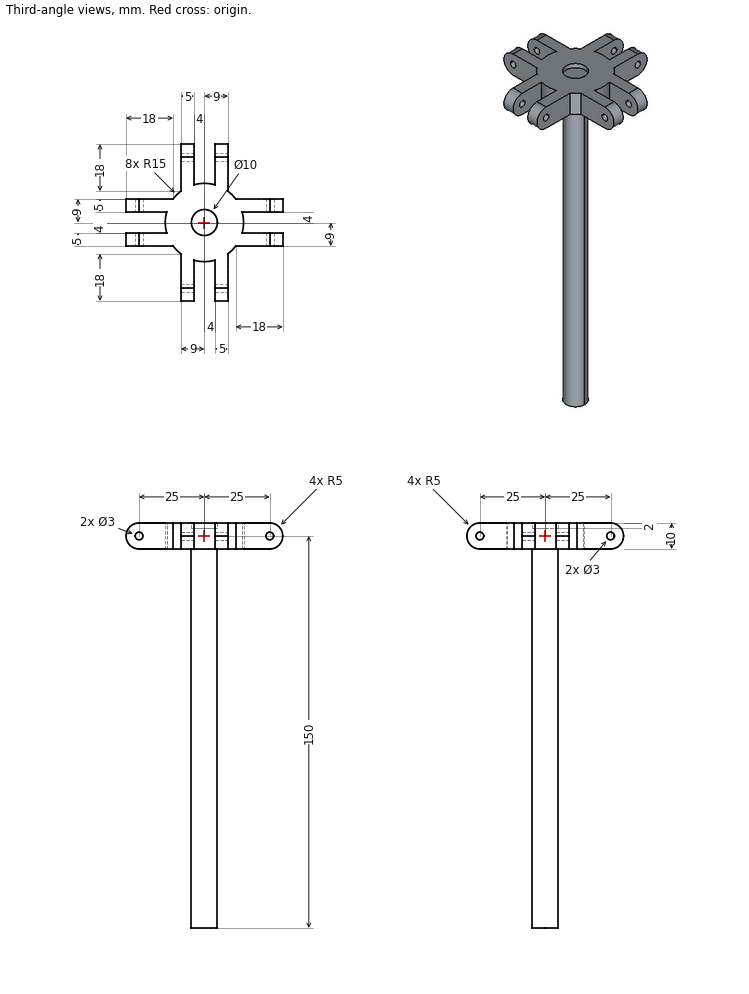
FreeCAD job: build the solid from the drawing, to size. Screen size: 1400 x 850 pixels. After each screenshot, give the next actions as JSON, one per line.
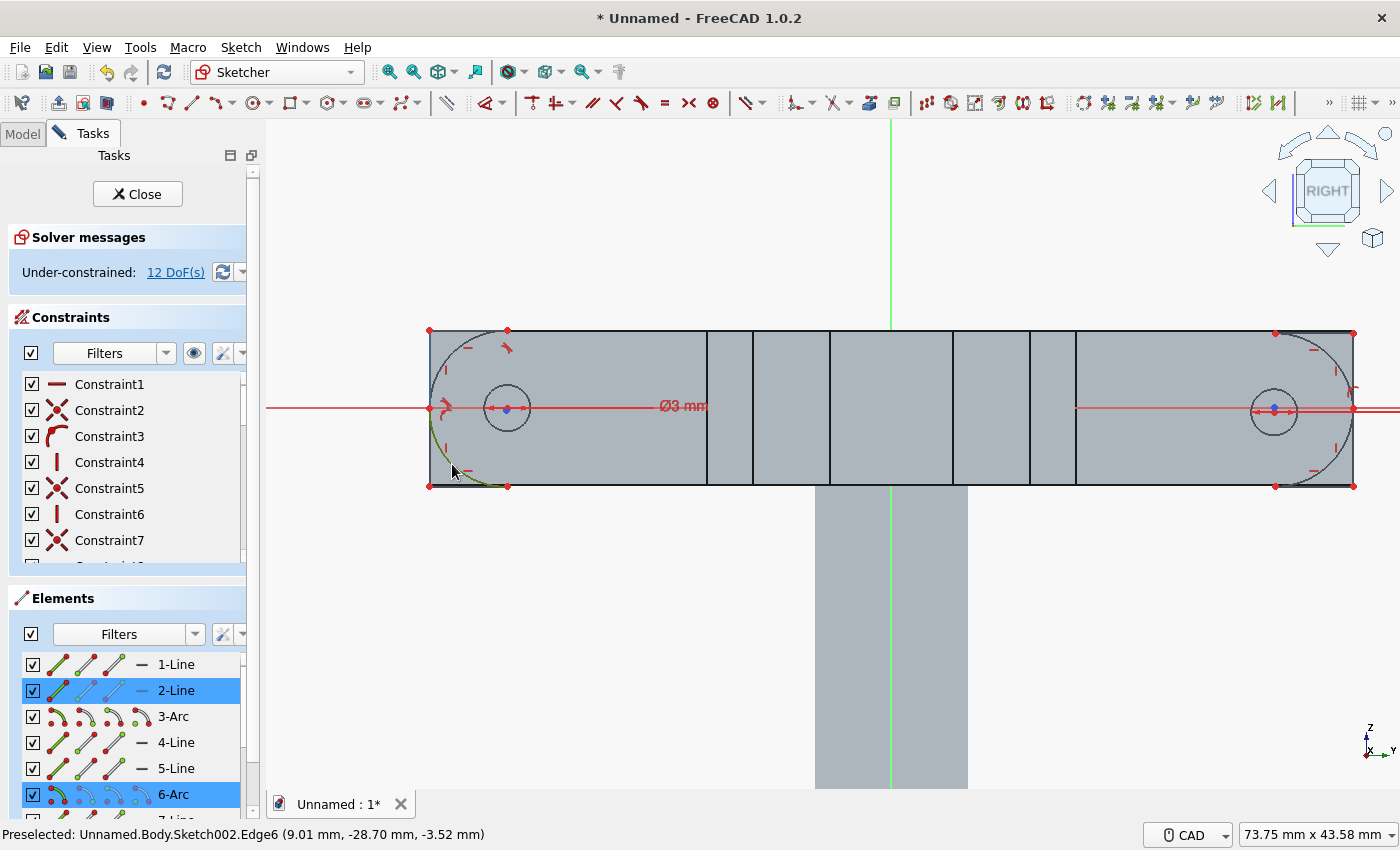
{"action": "key", "text": "t"}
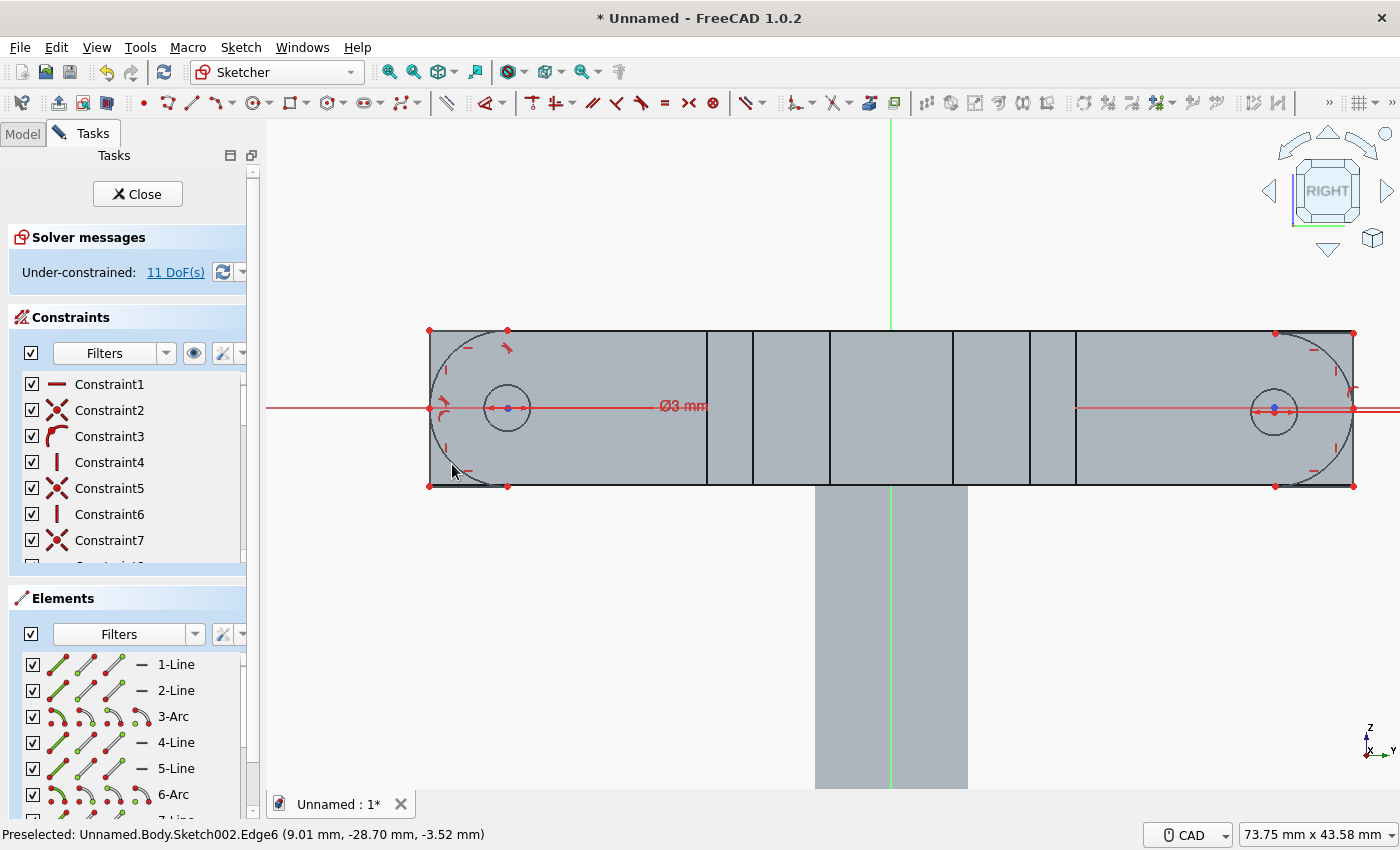
{"action": "left_click", "coordinate": [453, 487]}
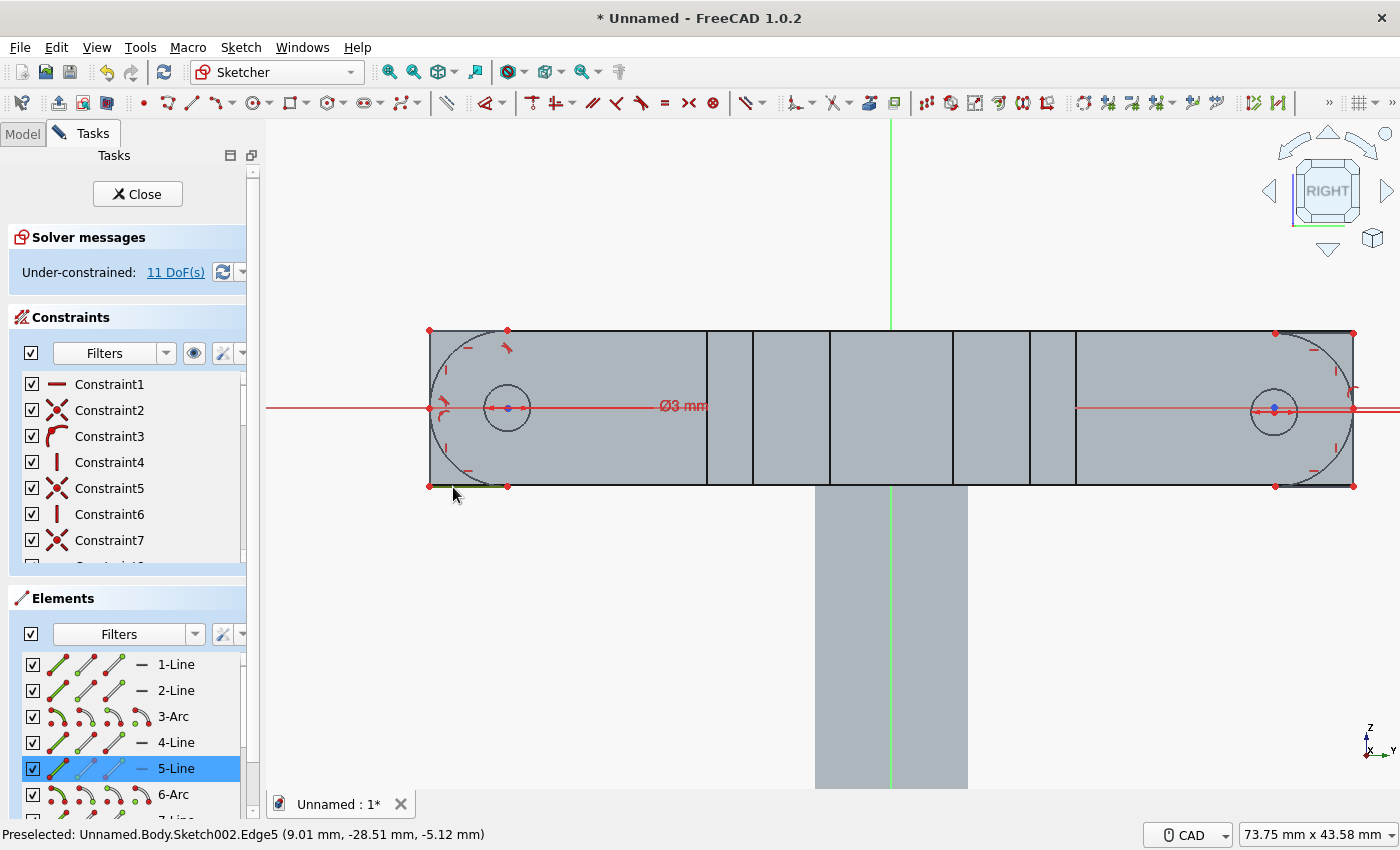
{"action": "left_click", "coordinate": [452, 463]}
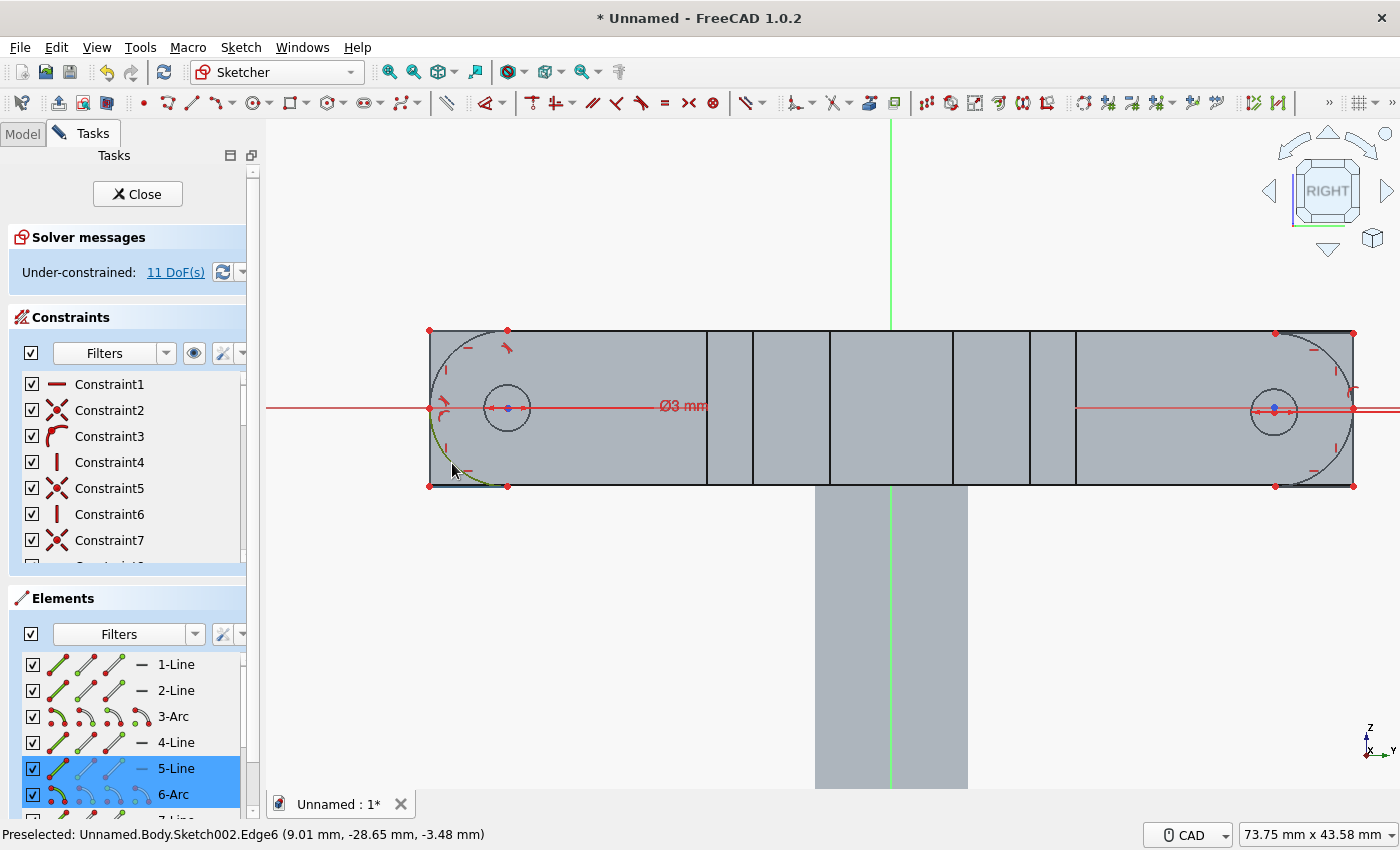
{"action": "left_click", "coordinate": [642, 104]}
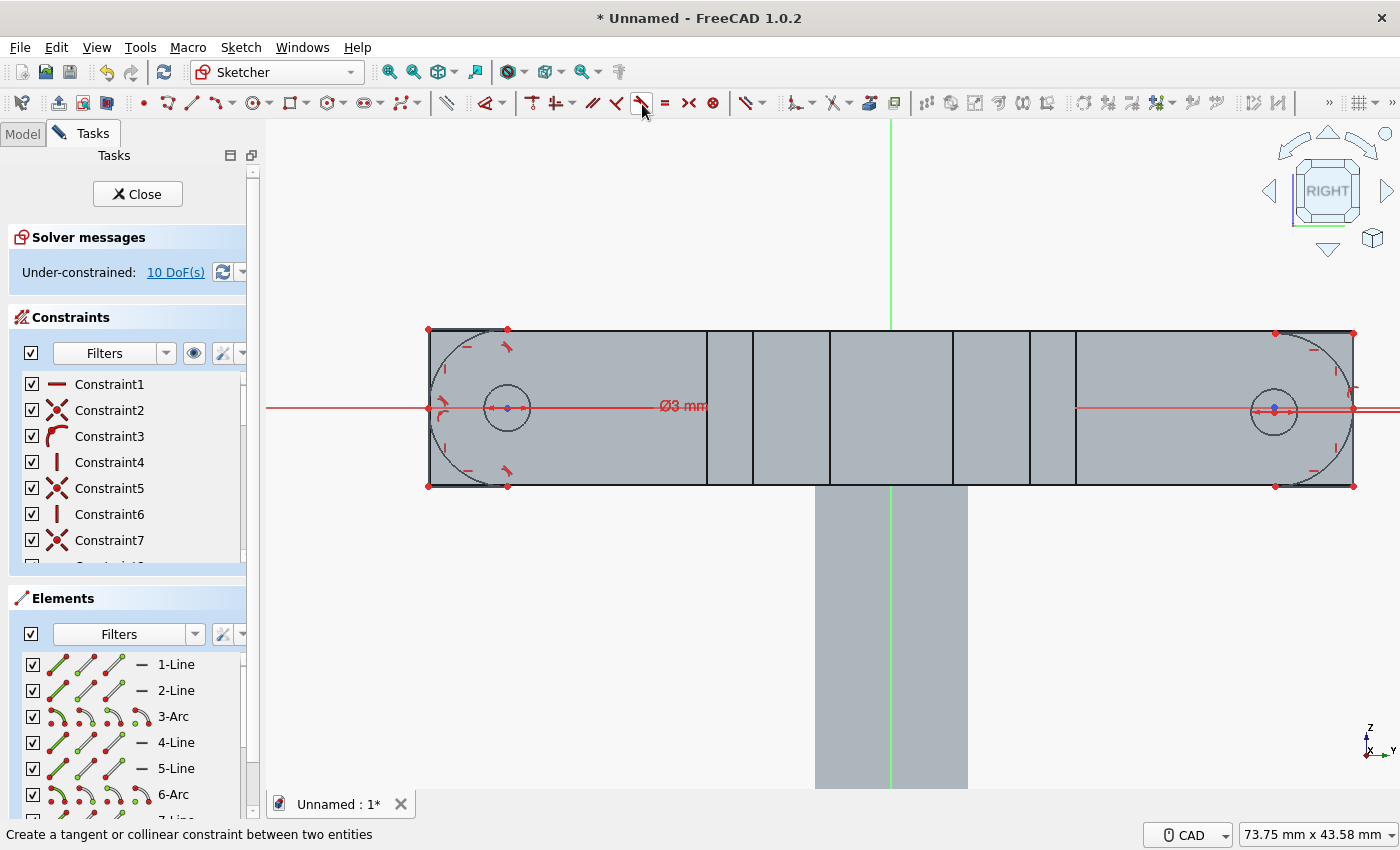
{"action": "scroll", "coordinate": [507, 547], "scroll_direction": "down", "scroll_amount": 2}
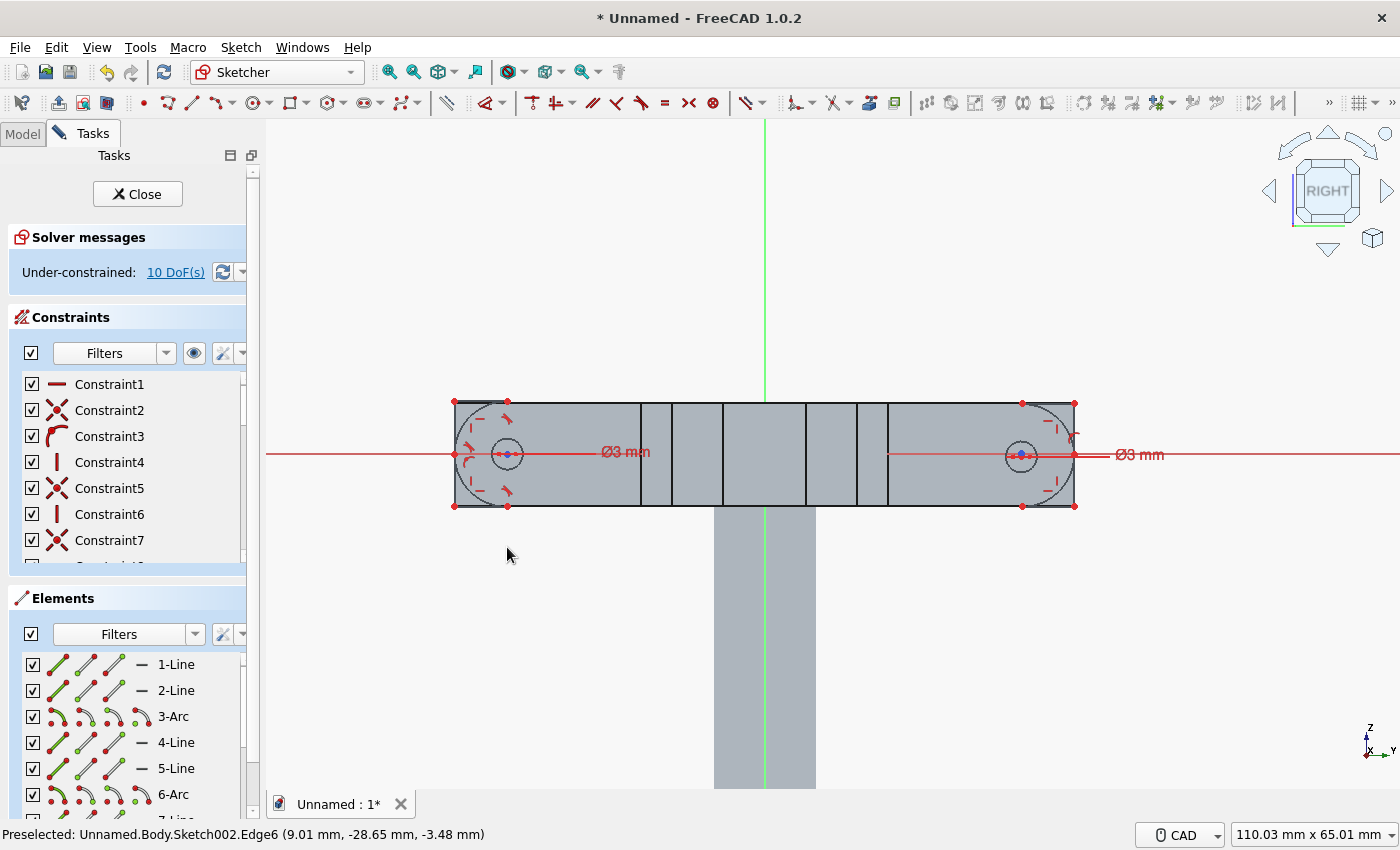
{"action": "left_click", "coordinate": [1074, 419]}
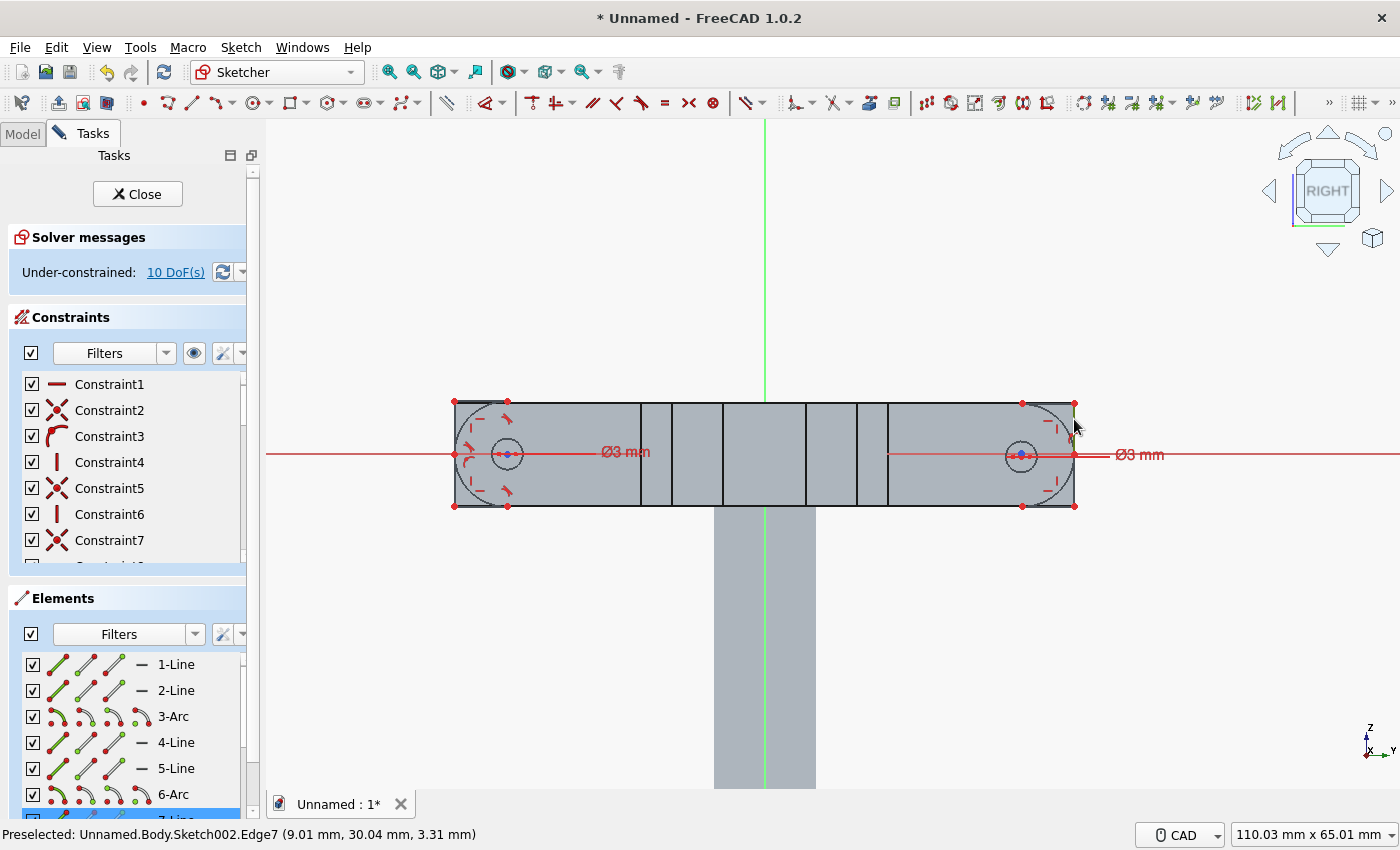
{"action": "left_click", "coordinate": [1058, 419]}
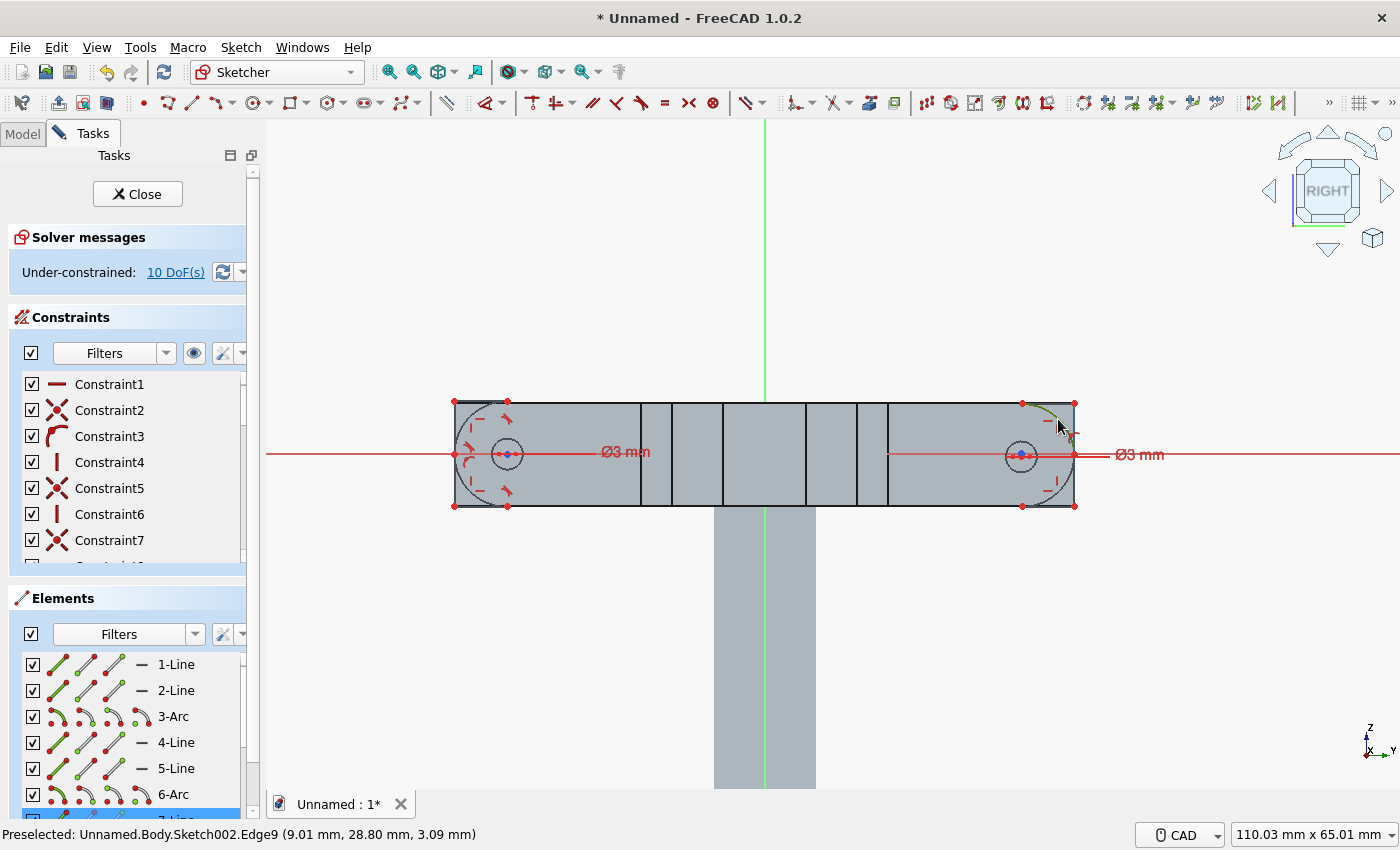
{"action": "key", "text": "t"}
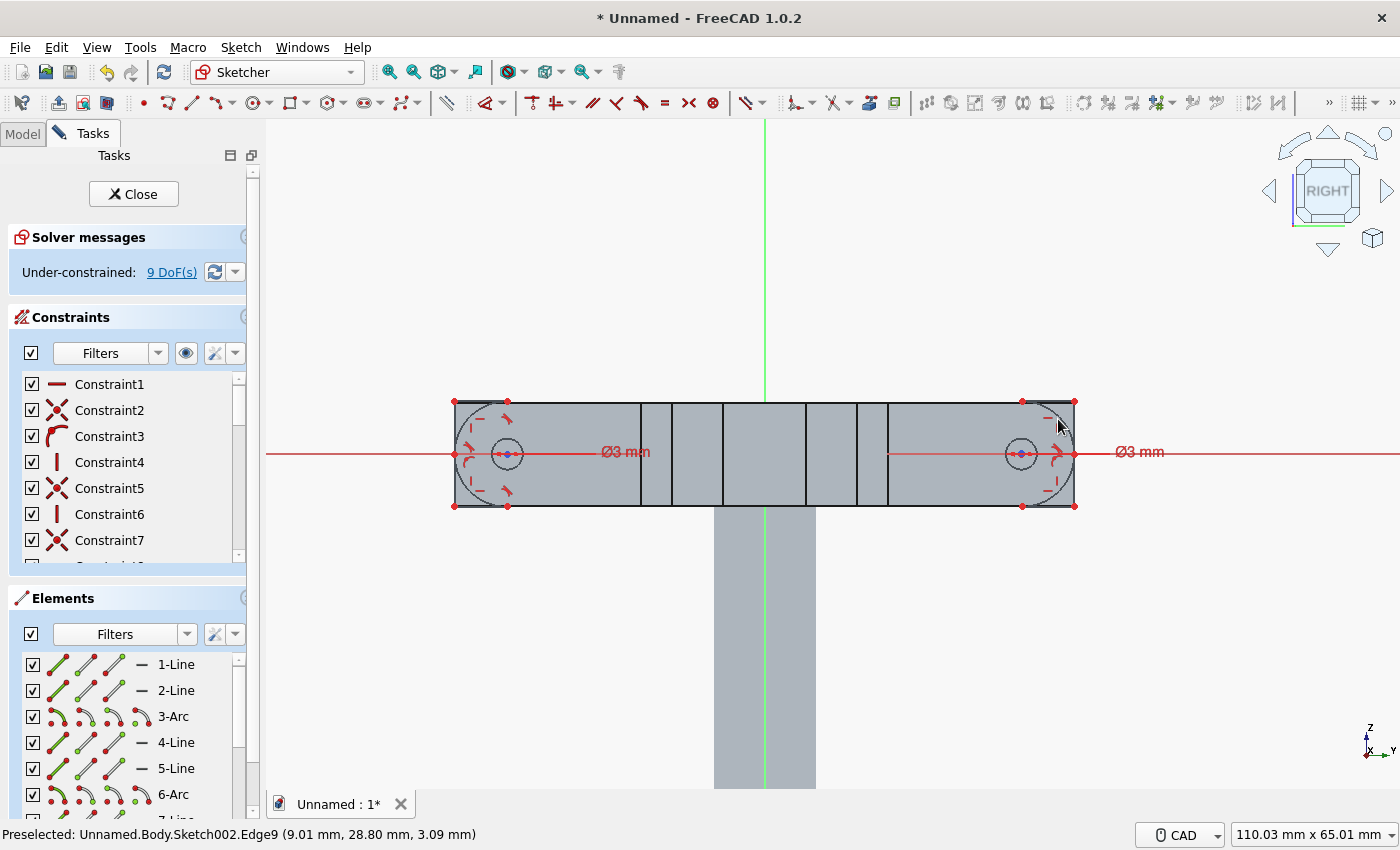
{"action": "left_click", "coordinate": [1074, 417]}